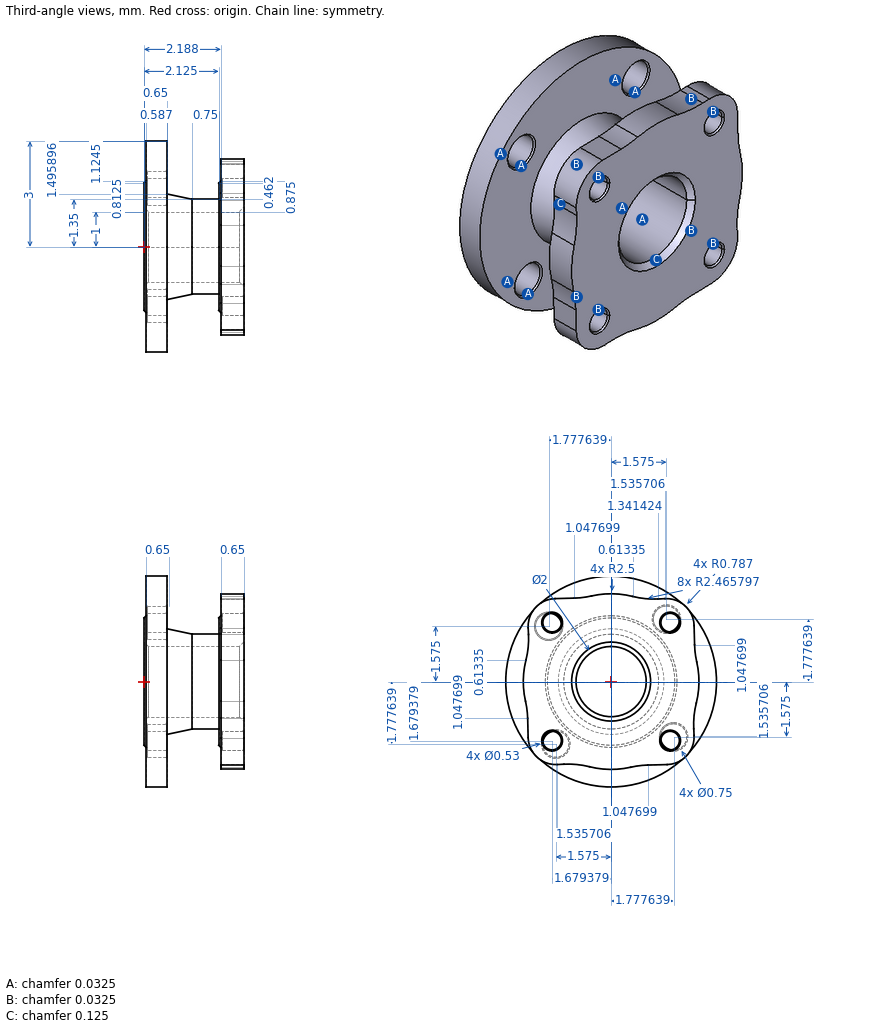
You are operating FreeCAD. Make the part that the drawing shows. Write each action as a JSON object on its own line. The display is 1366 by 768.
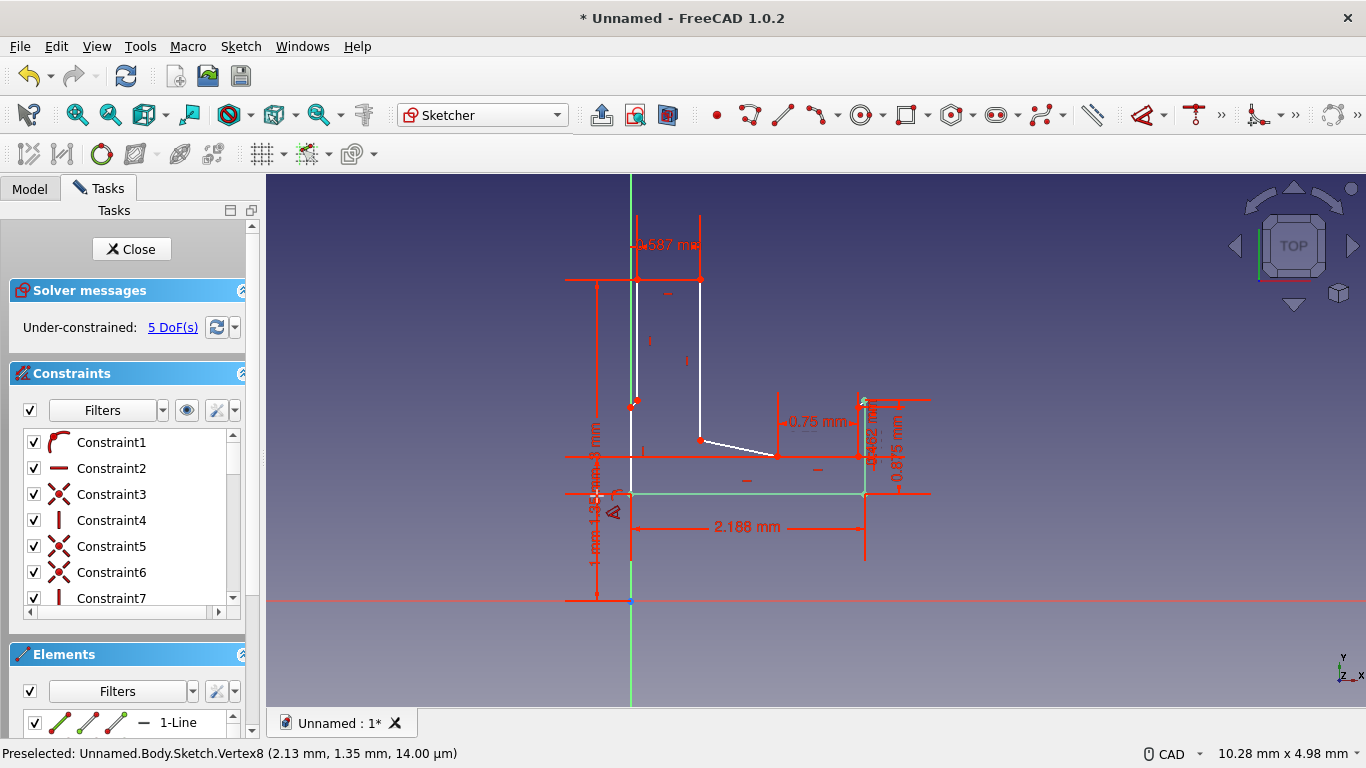
{"action": "left_click", "coordinate": [700, 440]}
{"action": "left_click", "coordinate": [665, 635]}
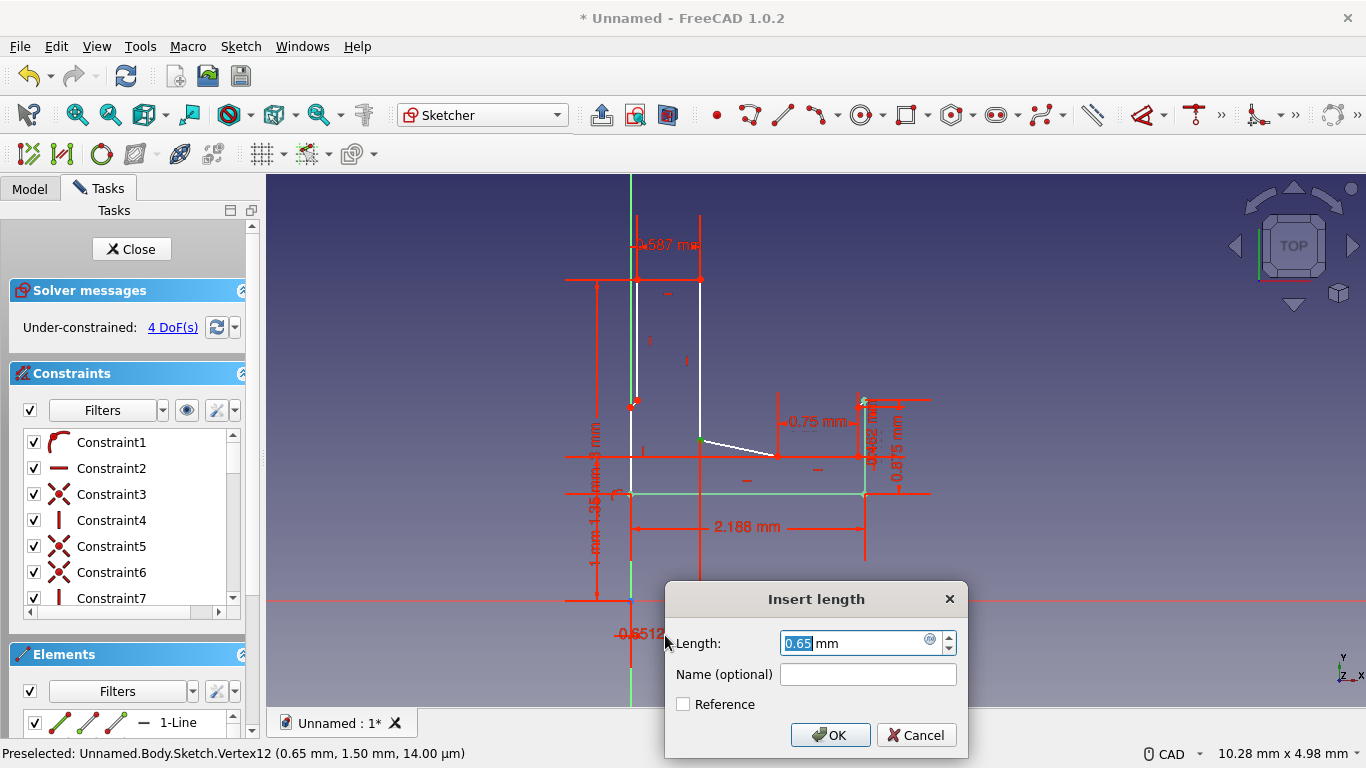
{"action": "type", "text": "0.65"}
{"action": "key", "text": "Return"}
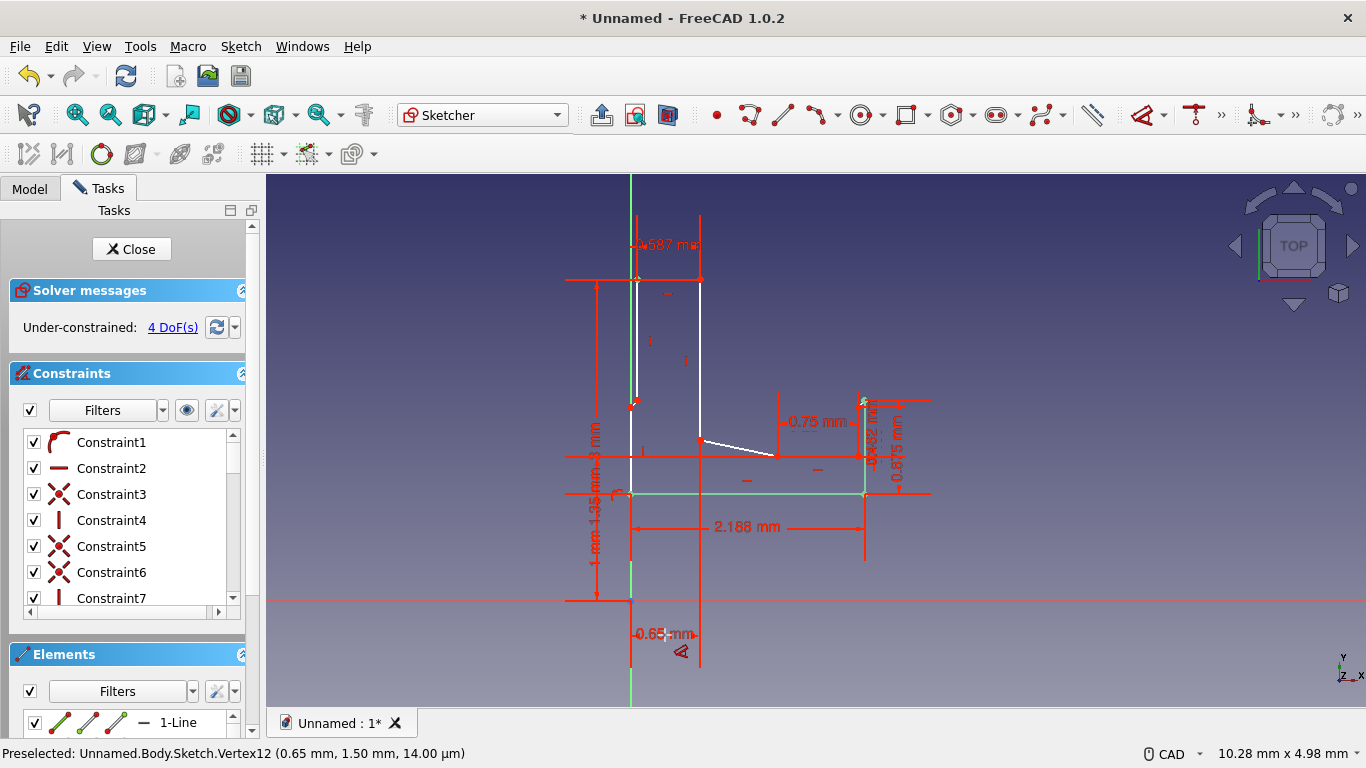
{"action": "scroll", "coordinate": [637, 316], "scroll_direction": "up", "scroll_amount": 4}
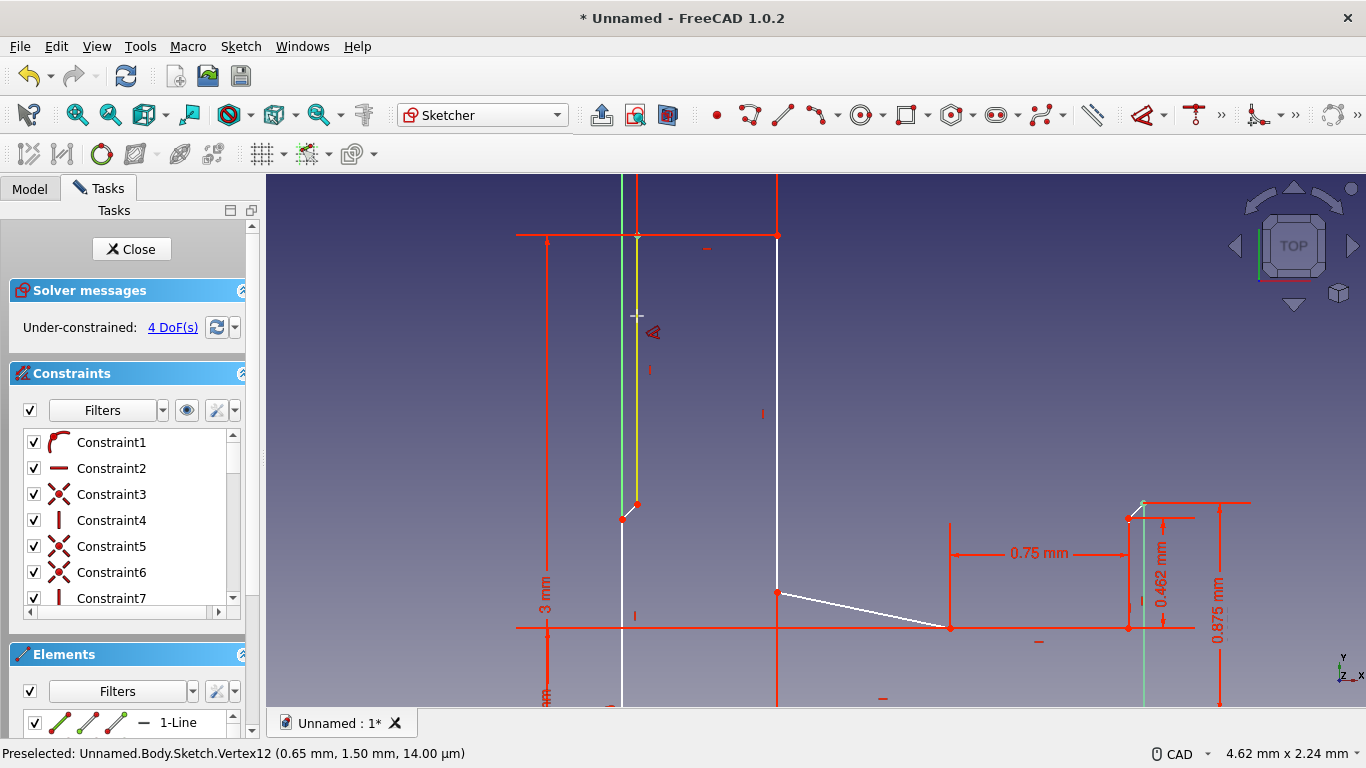
{"action": "left_click", "coordinate": [637, 316]}
{"action": "left_click", "coordinate": [603, 370]}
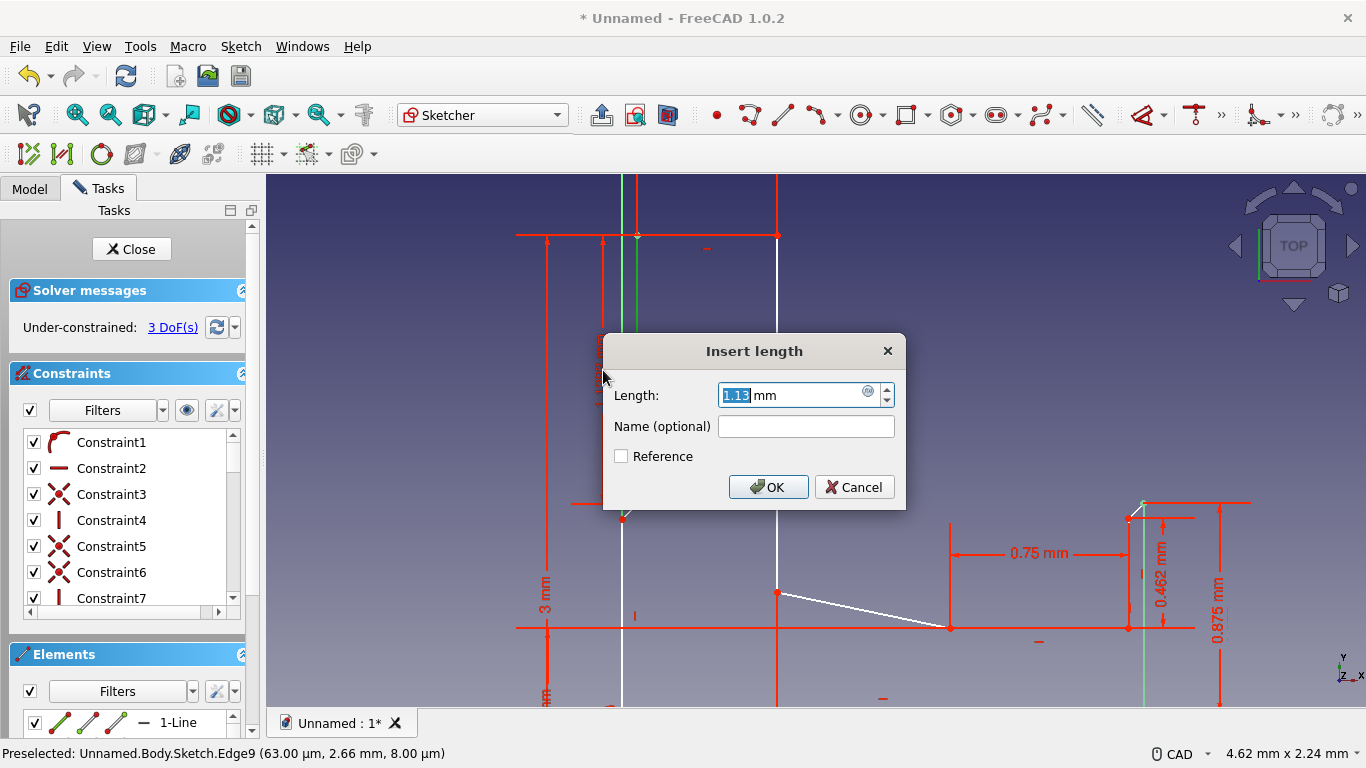
{"action": "type", "text": "1.1245"}
{"action": "key", "text": "Return"}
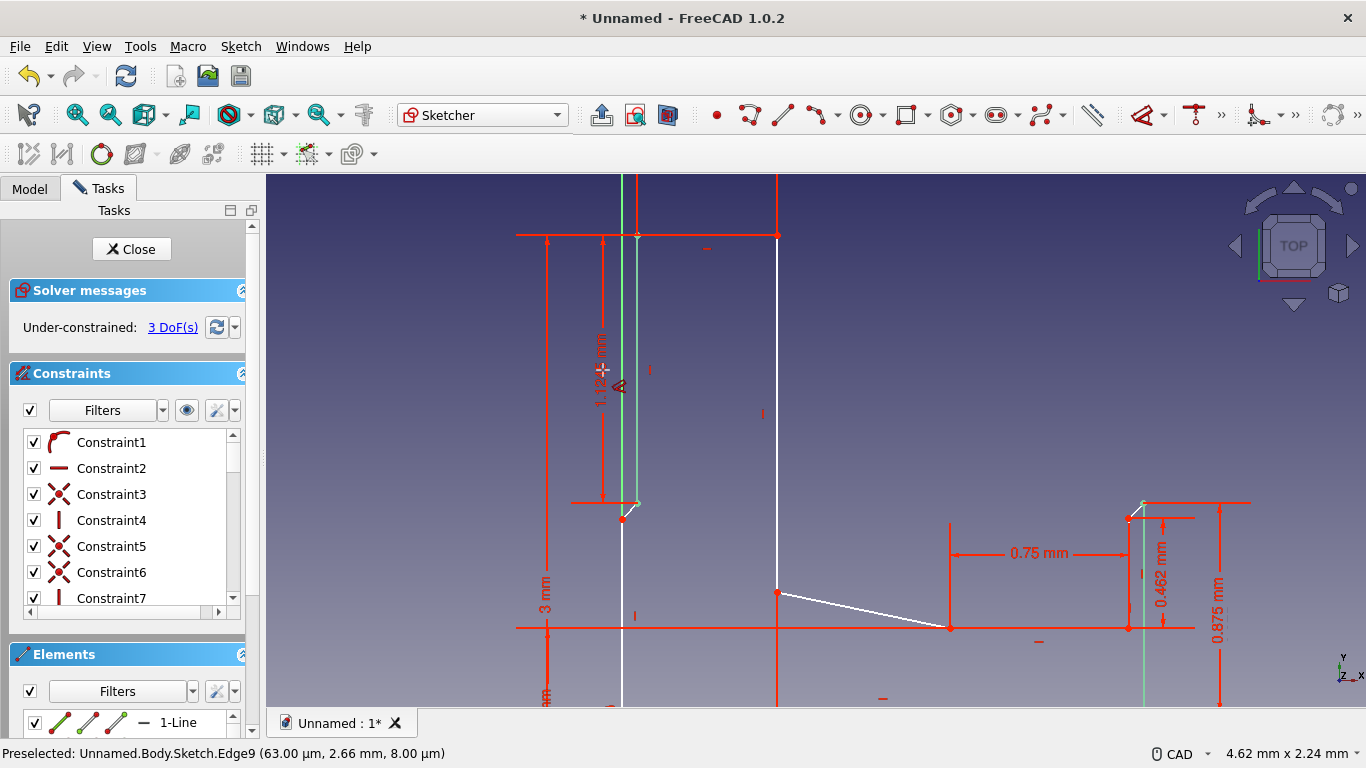
{"action": "left_click", "coordinate": [622, 577]}
{"action": "left_click", "coordinate": [588, 562]}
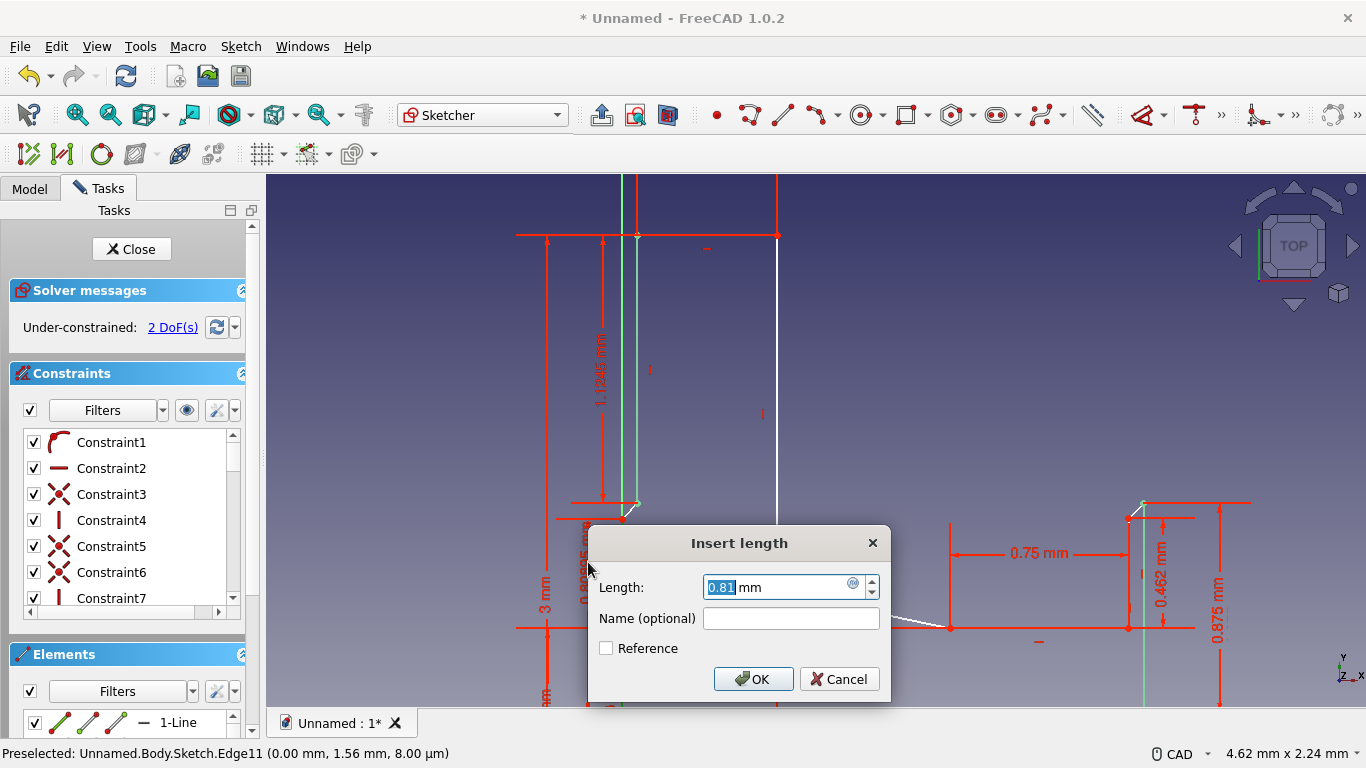
{"action": "type", "text": "0.8125"}
{"action": "key", "text": "Return"}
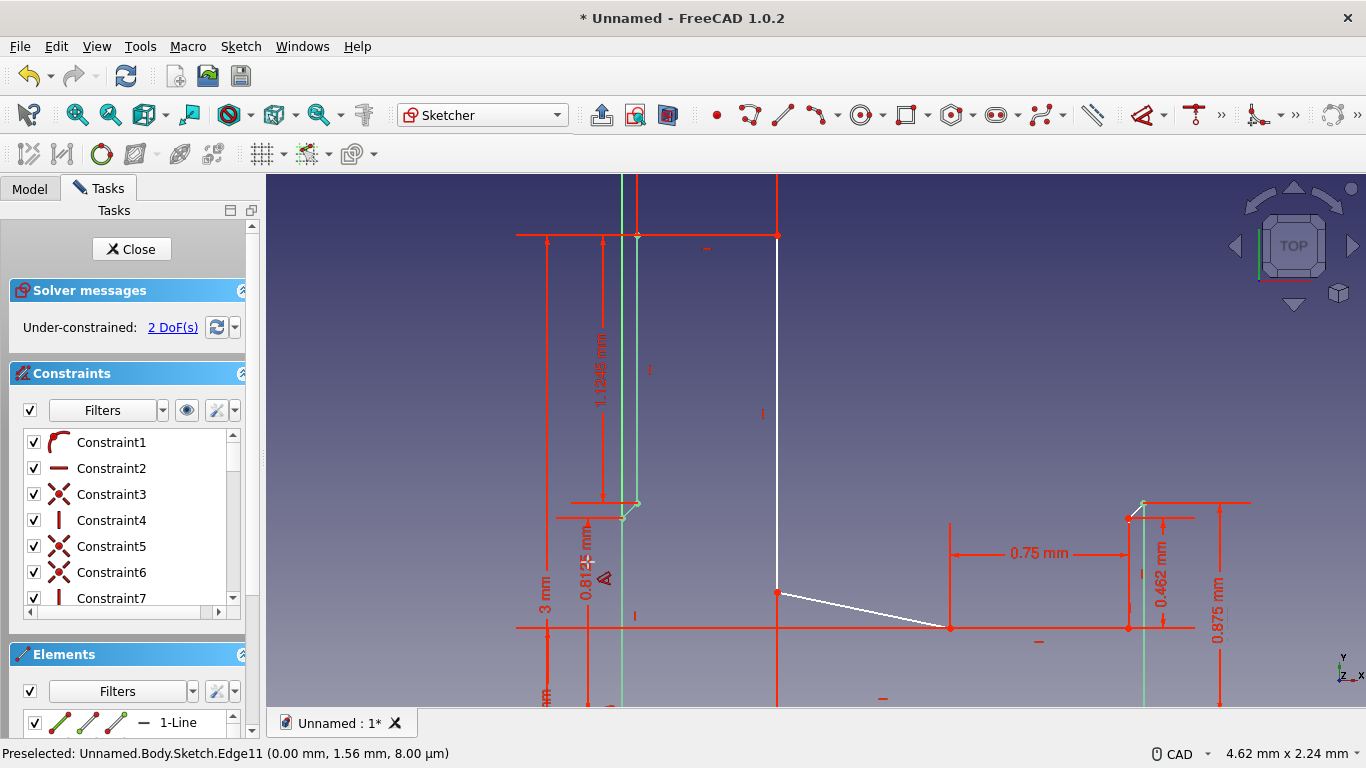
{"action": "left_click", "coordinate": [1129, 518]}
{"action": "left_click", "coordinate": [876, 484]}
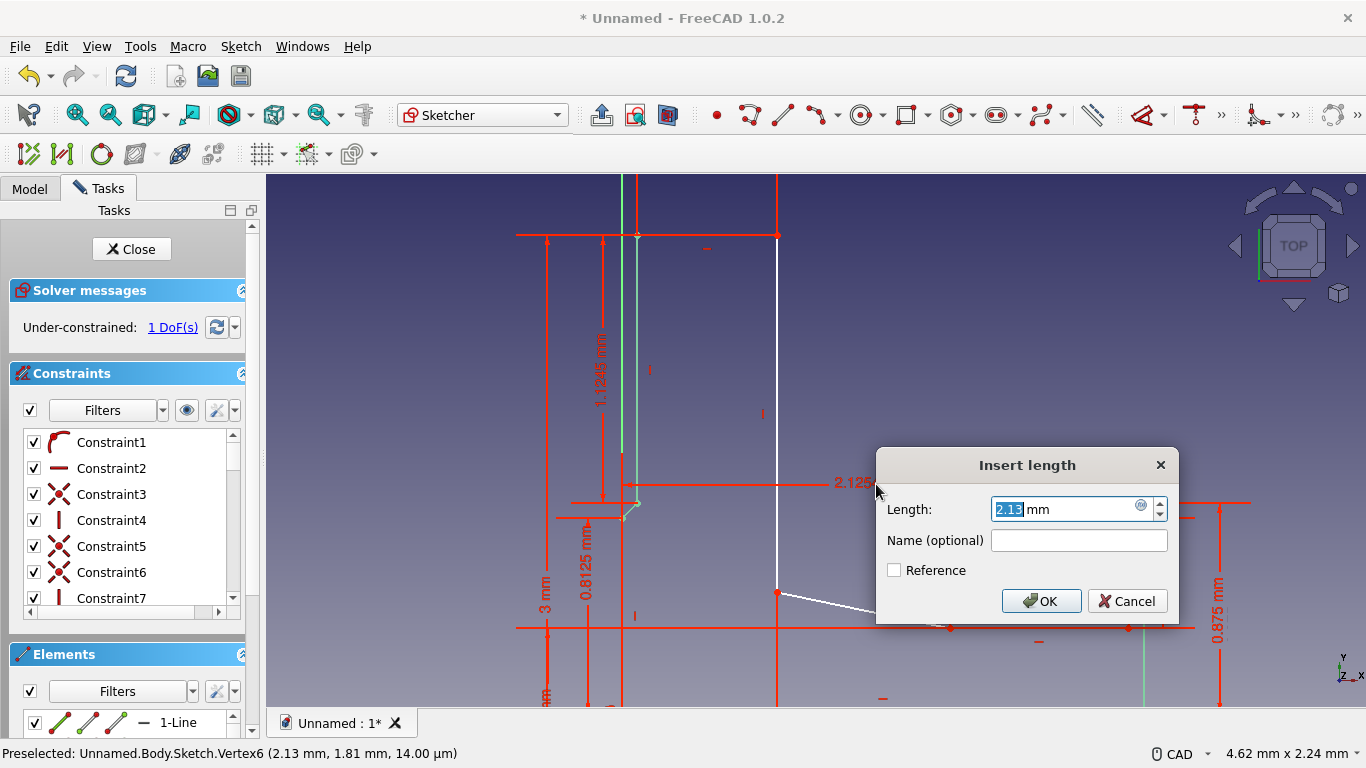
{"action": "type", "text": "2.125"}
{"action": "key", "text": "Return"}